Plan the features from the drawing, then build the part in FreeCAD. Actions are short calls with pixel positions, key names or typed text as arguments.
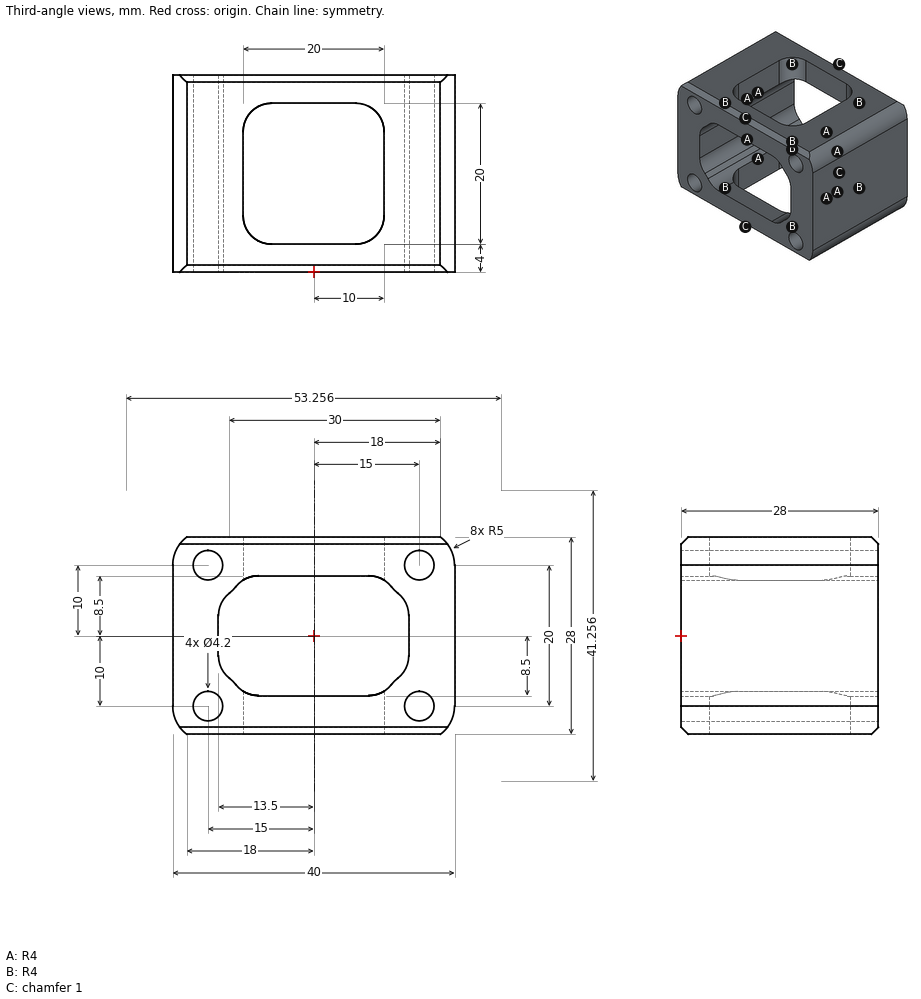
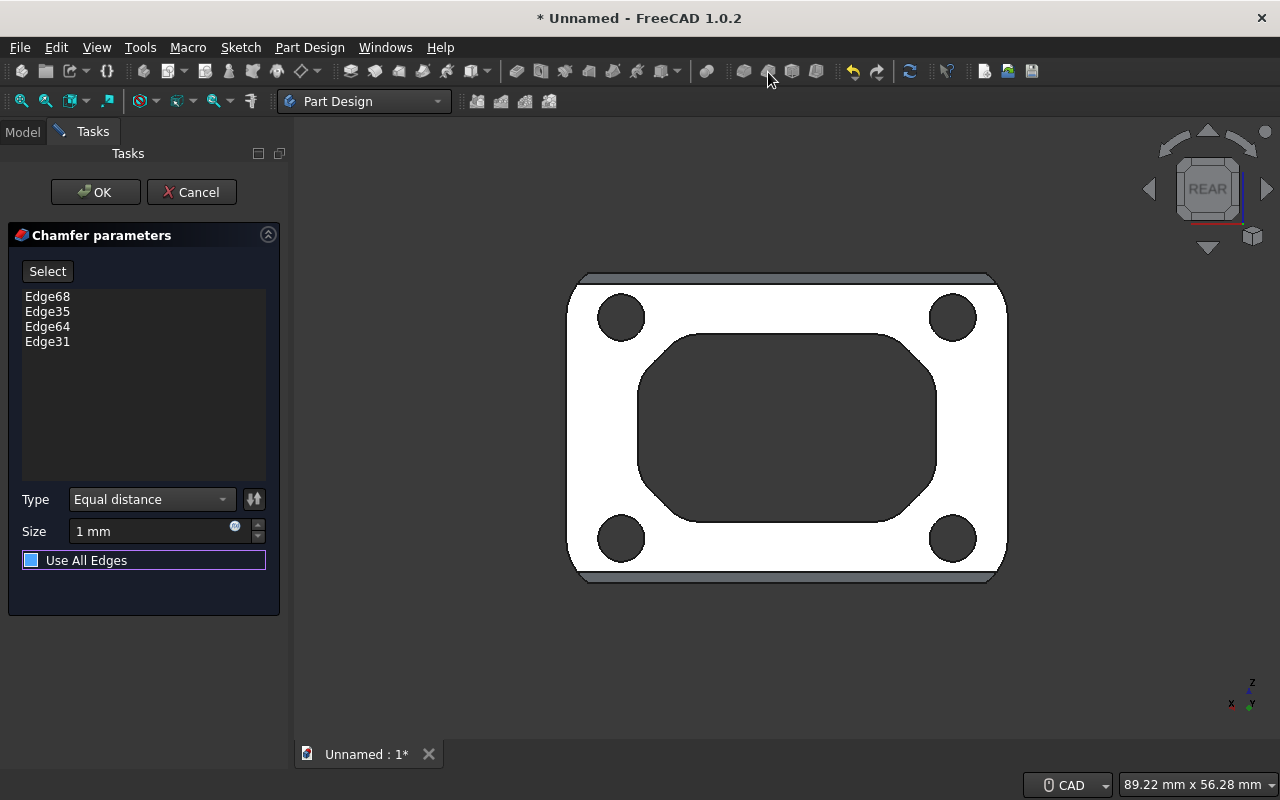
click(96, 192)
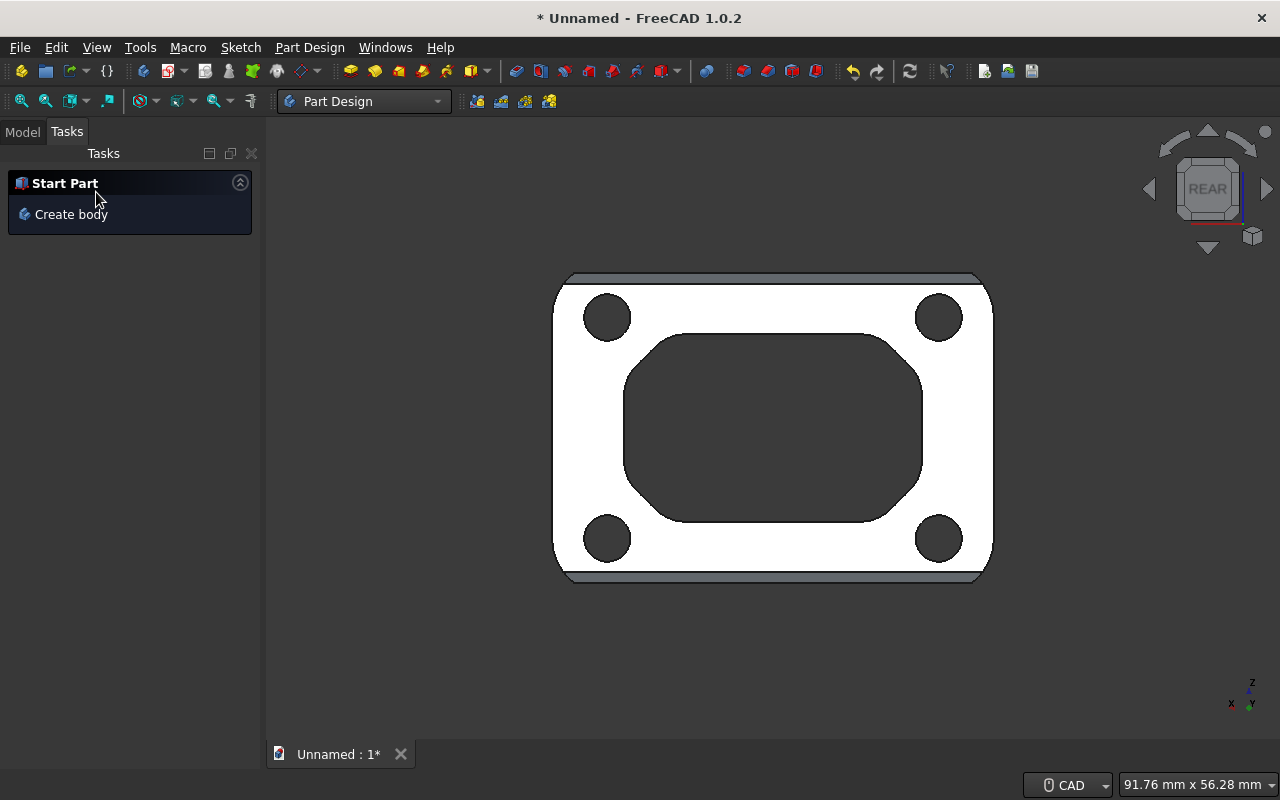
key(0)